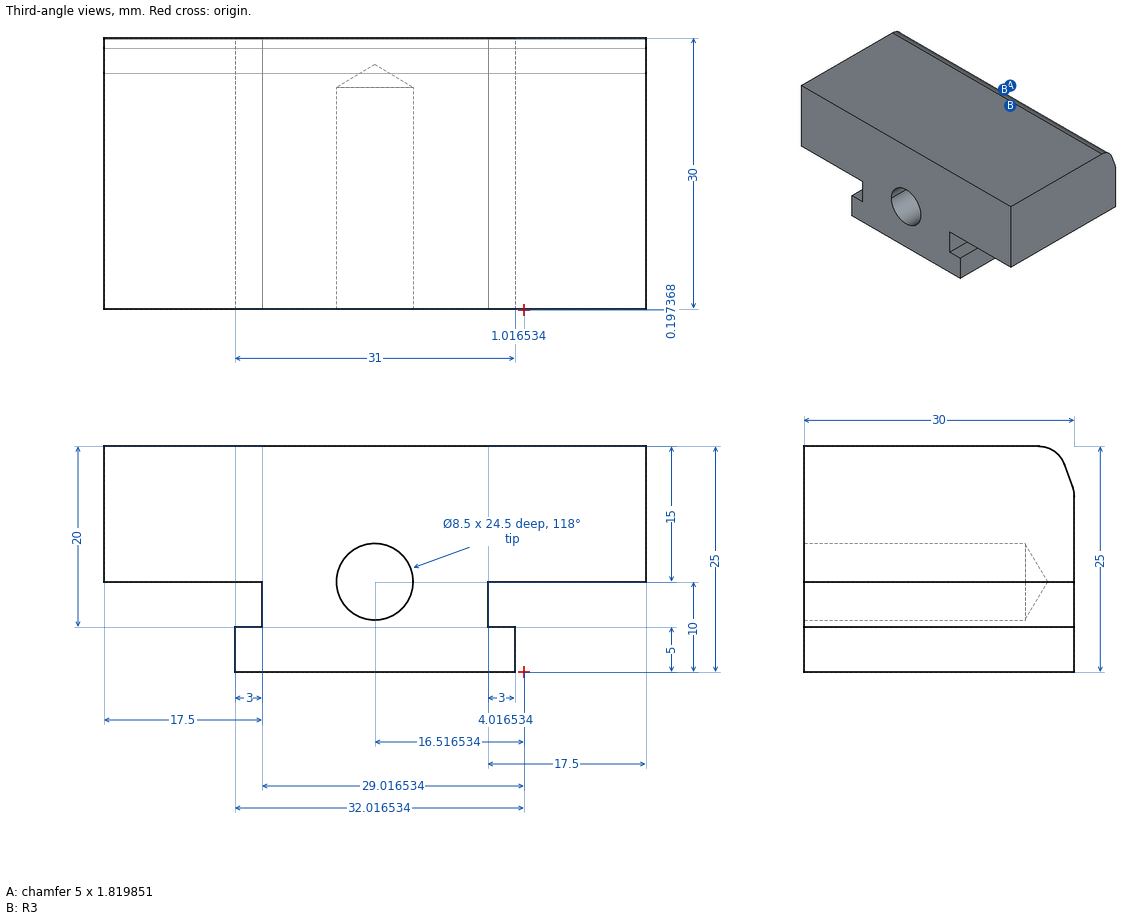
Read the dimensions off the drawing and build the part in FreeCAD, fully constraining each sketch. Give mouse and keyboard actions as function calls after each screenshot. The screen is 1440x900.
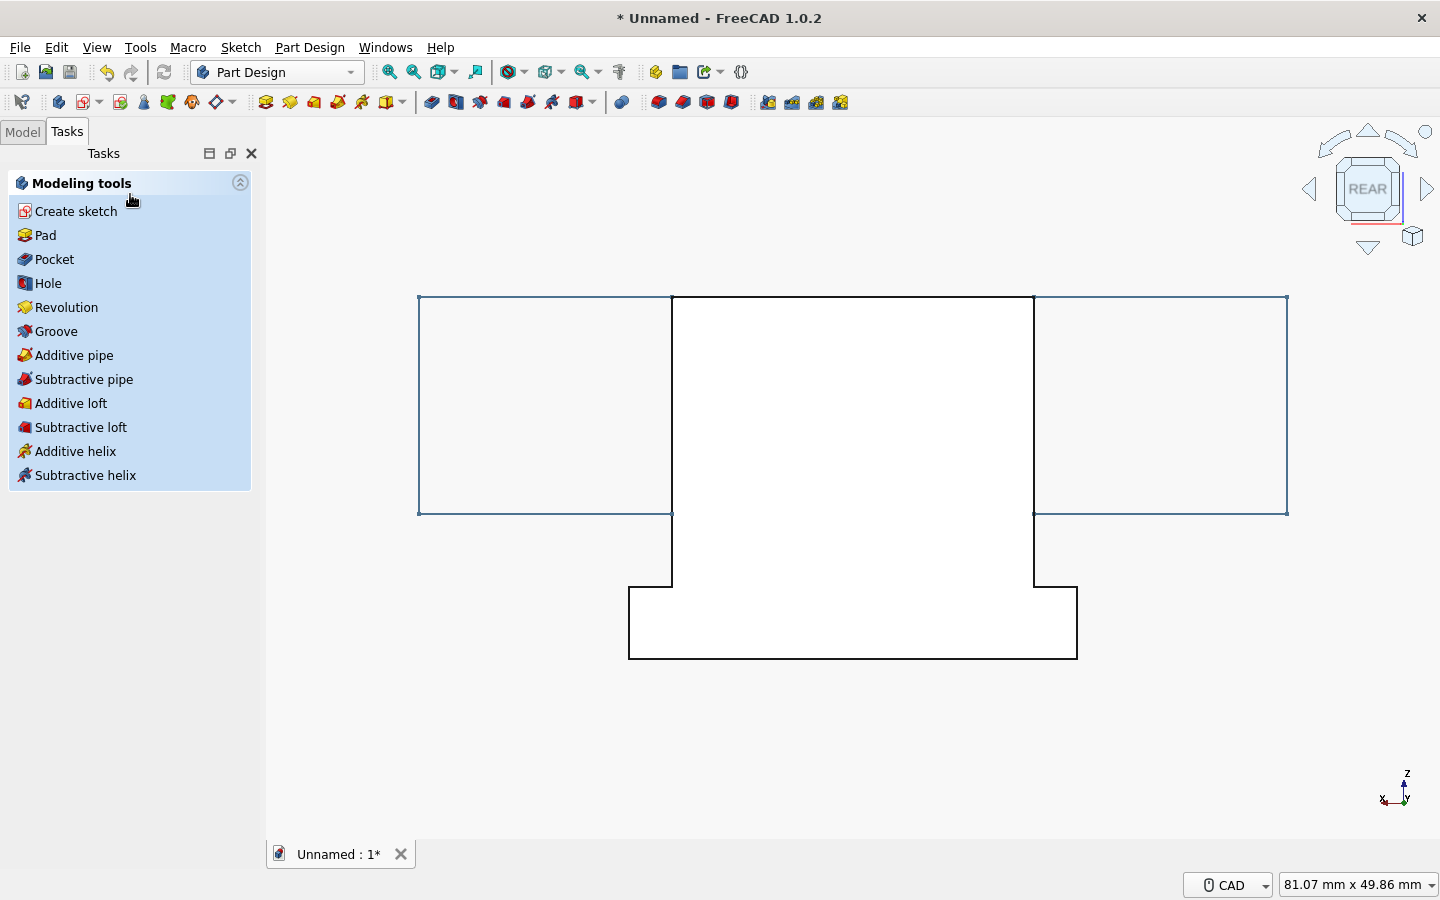
click(266, 102)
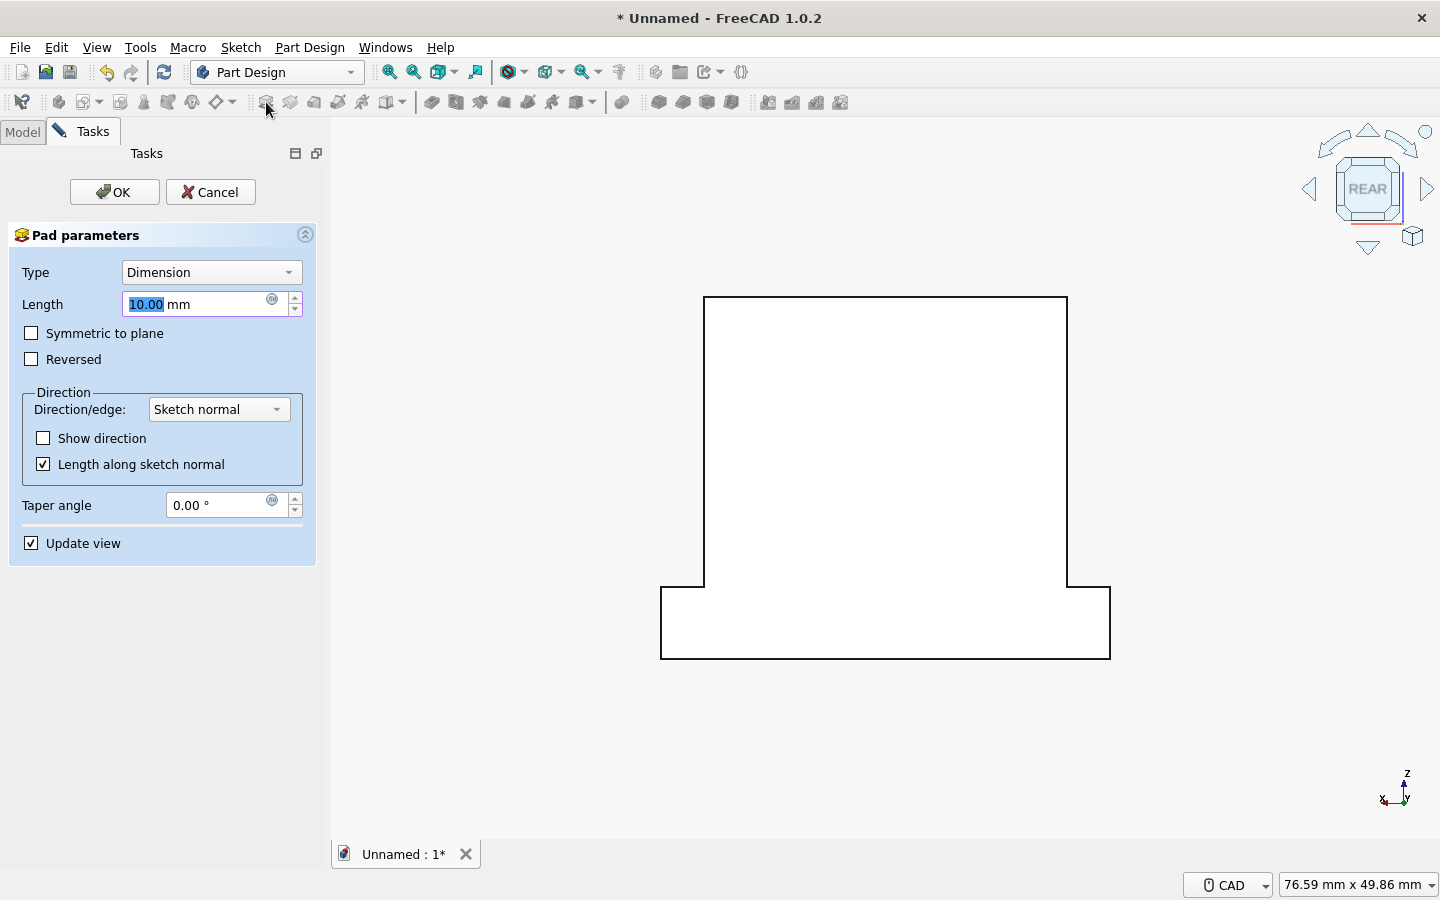
text(30)
key(Tab)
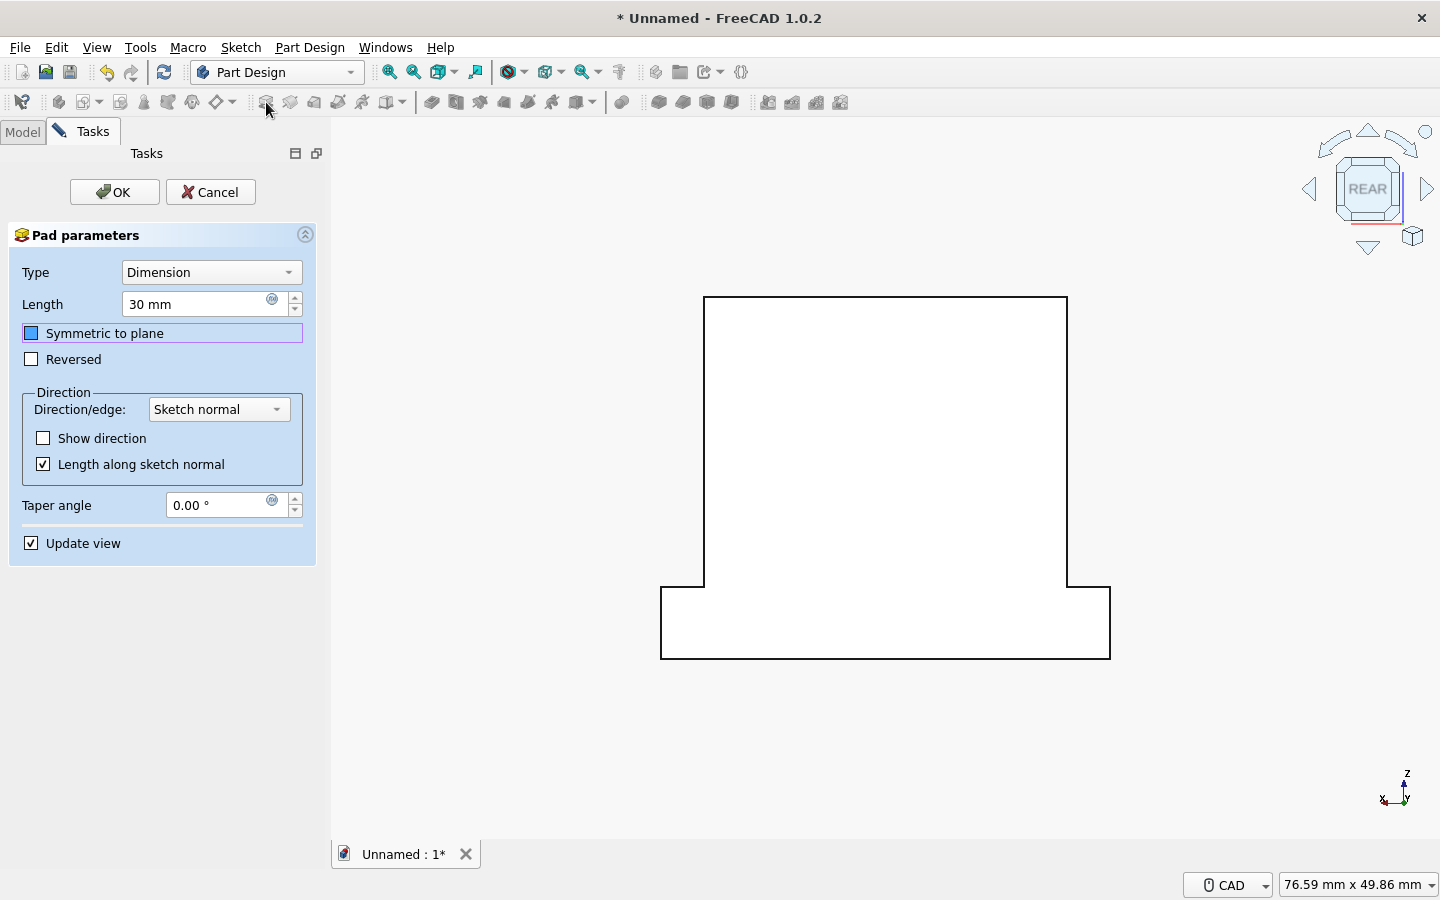
click(30, 359)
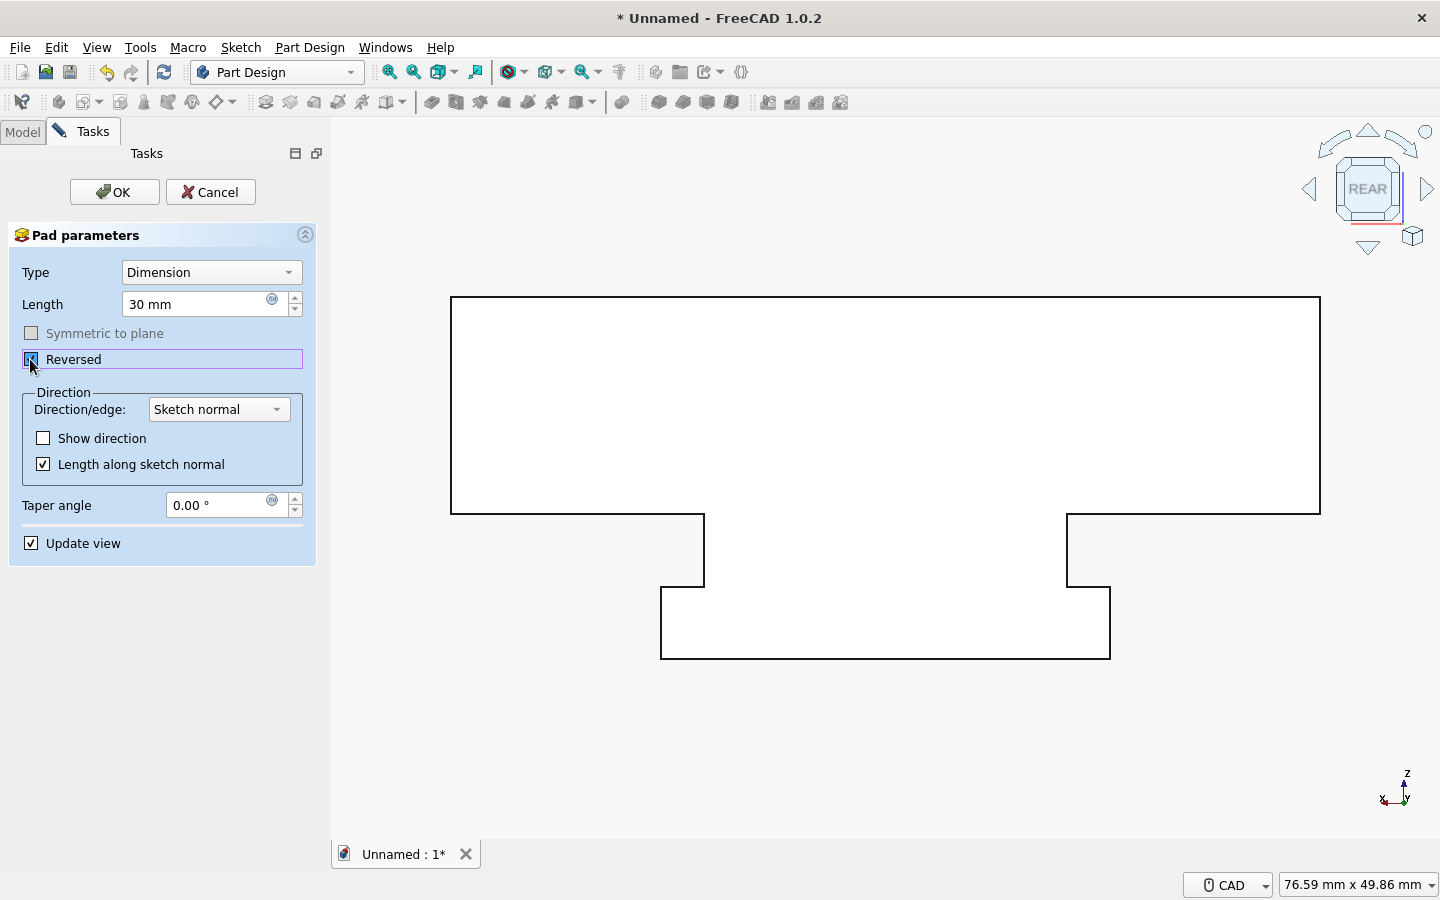
click(115, 192)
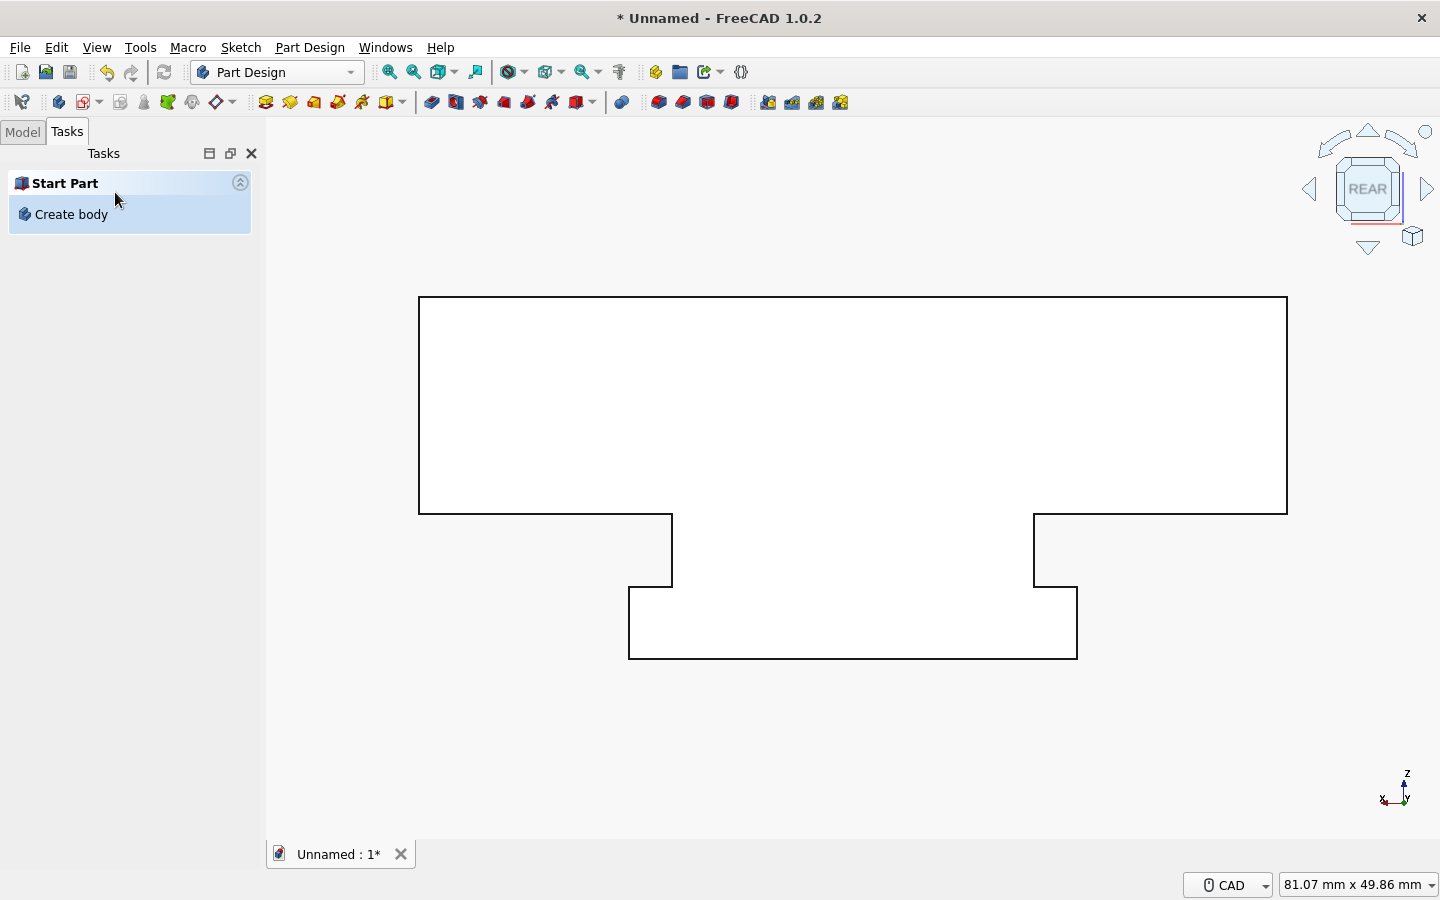
click(853, 296)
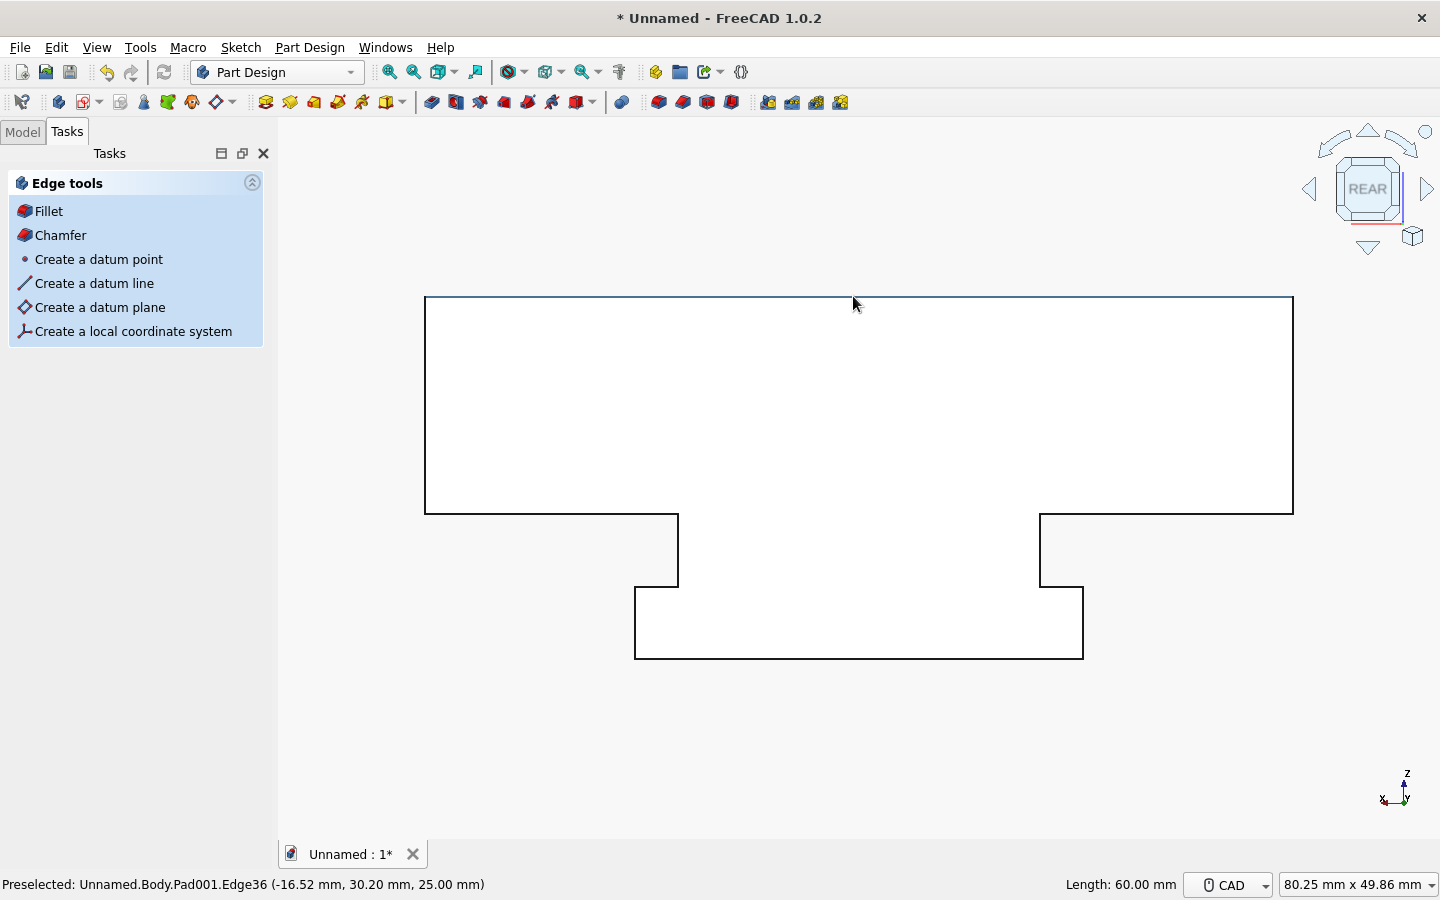
click(684, 102)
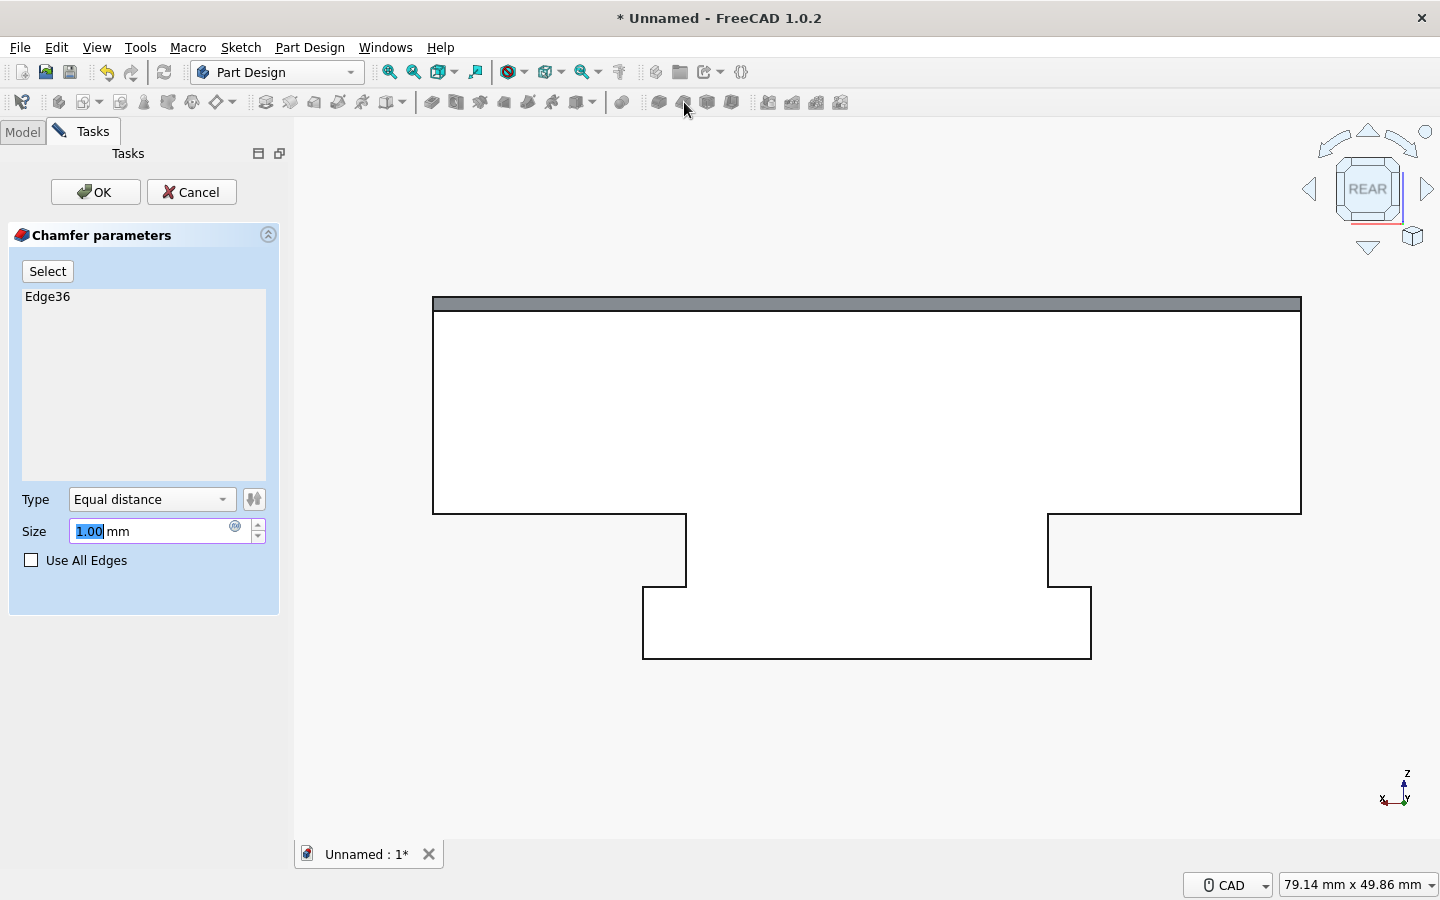
text(5)
key(Tab)